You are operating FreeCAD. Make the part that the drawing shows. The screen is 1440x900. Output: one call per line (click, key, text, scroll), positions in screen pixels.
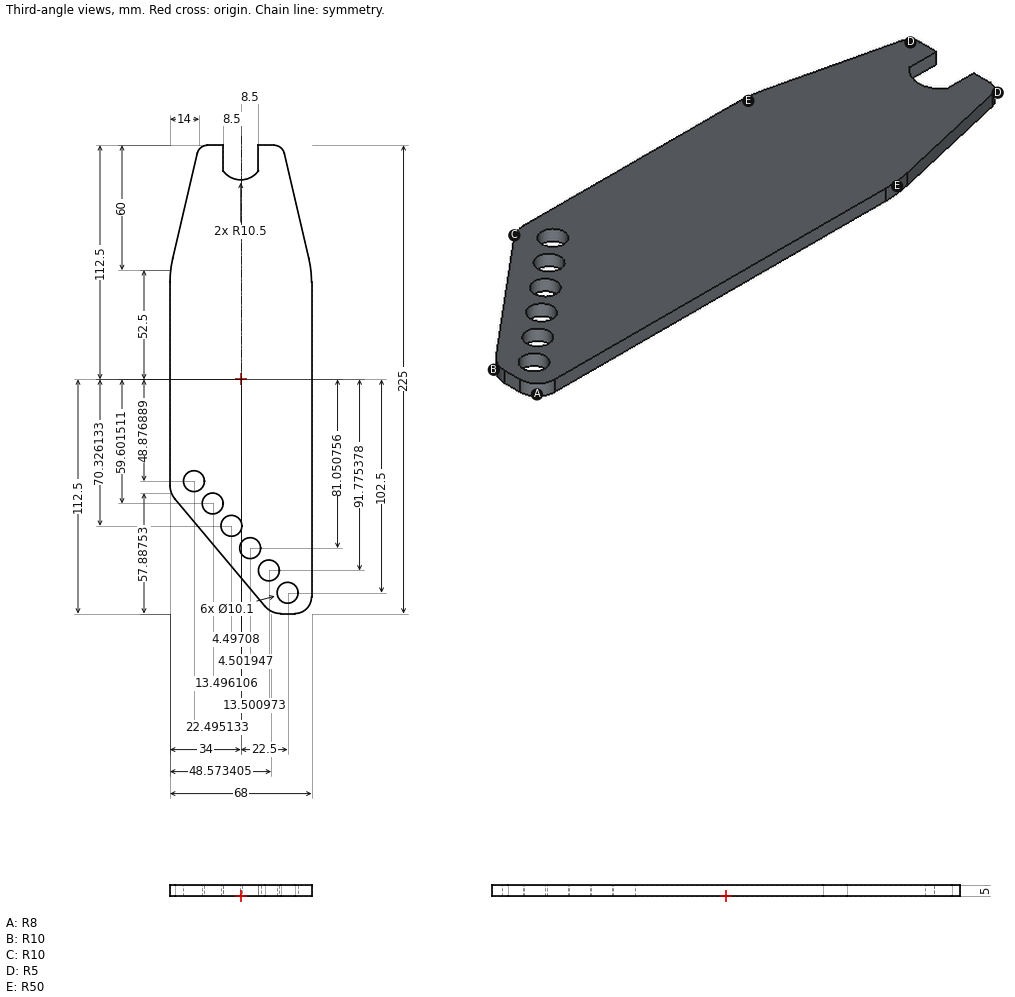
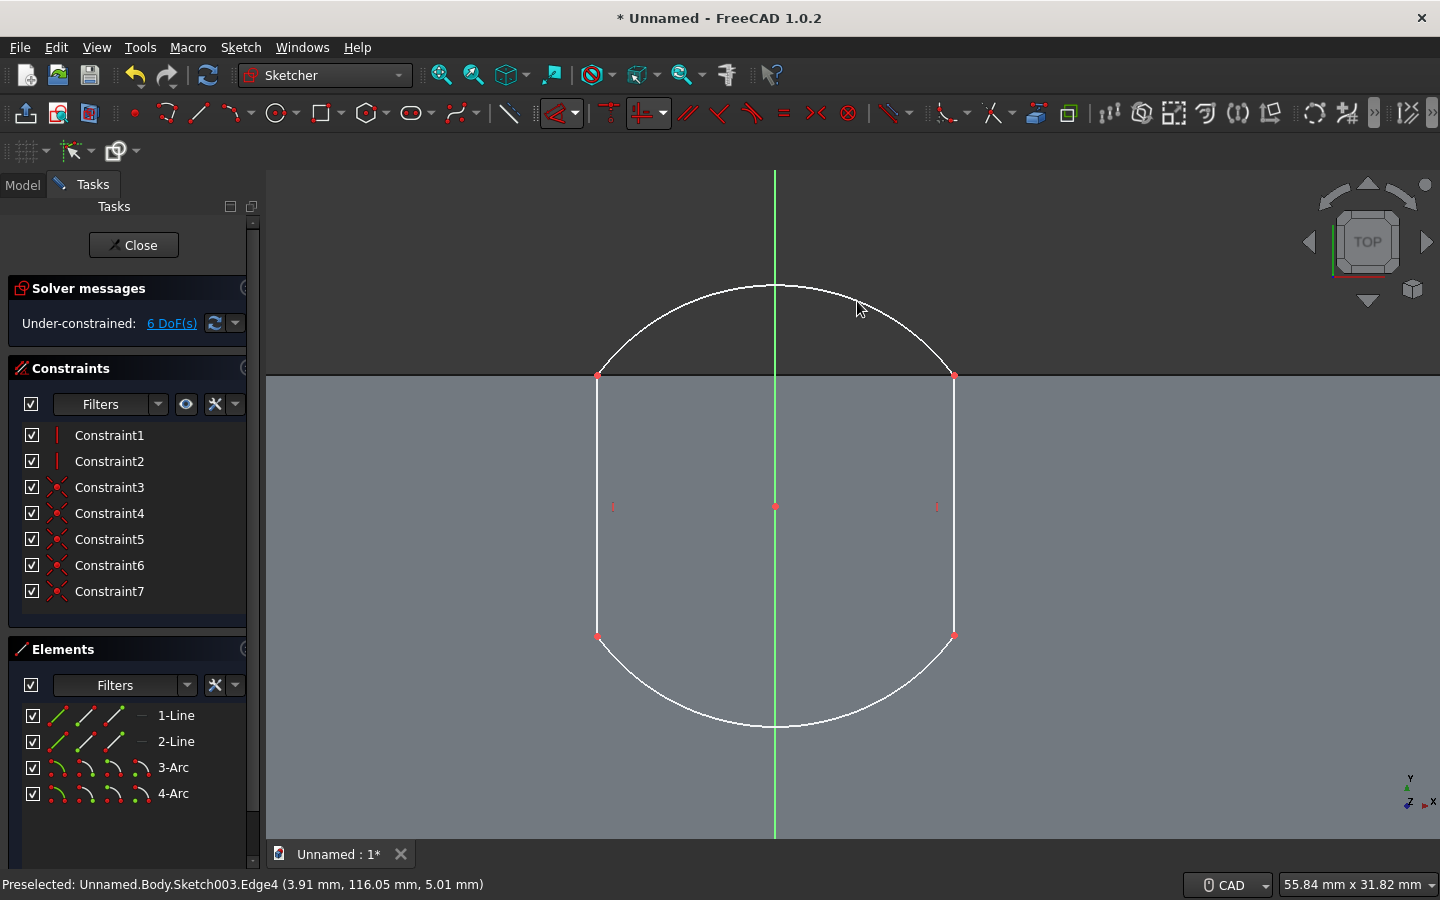
click(694, 711)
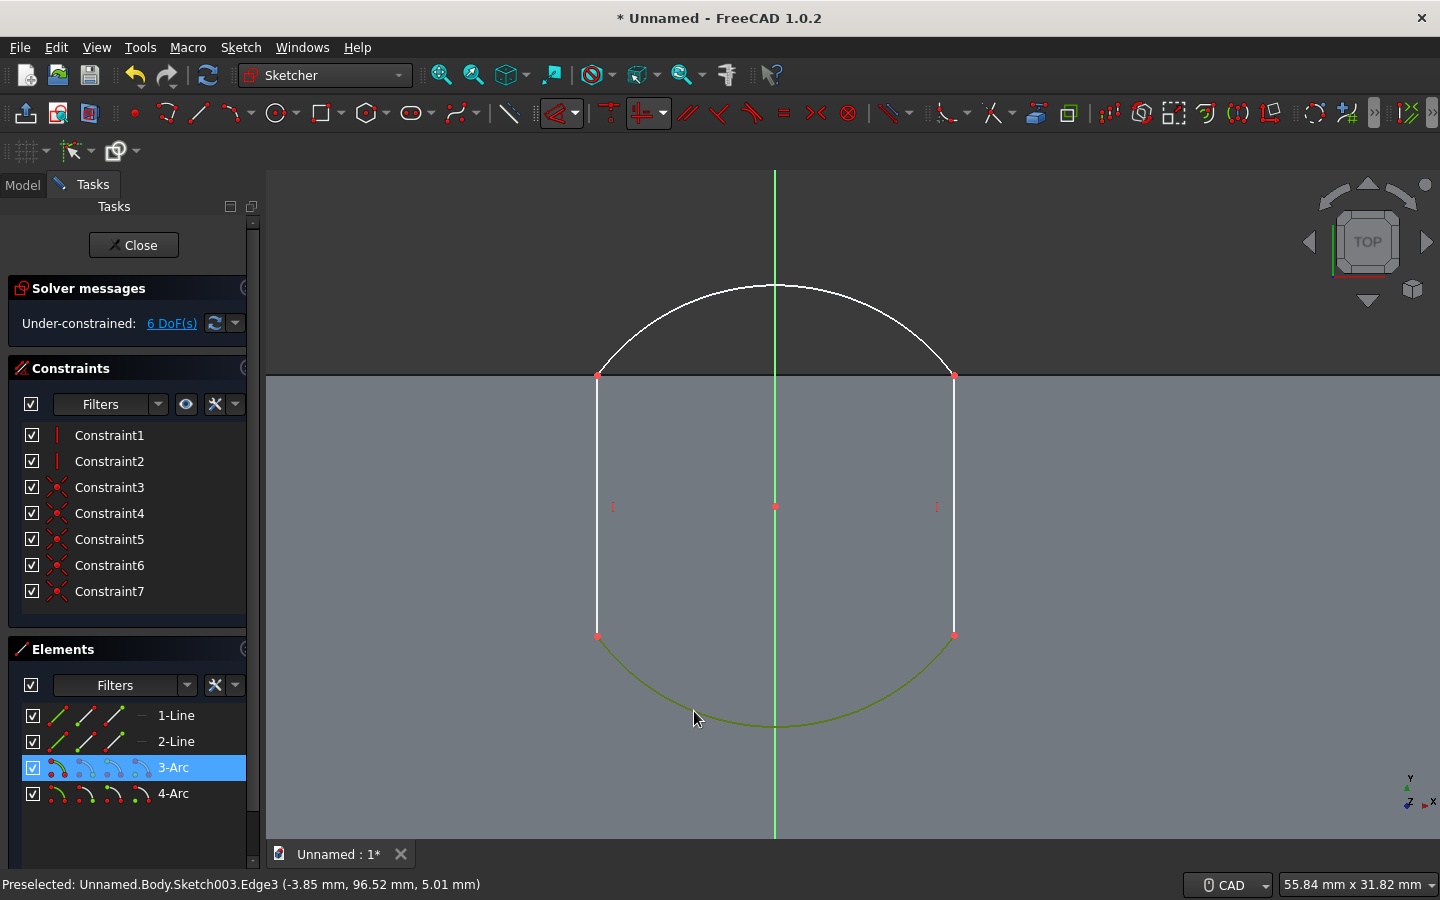
click(857, 301)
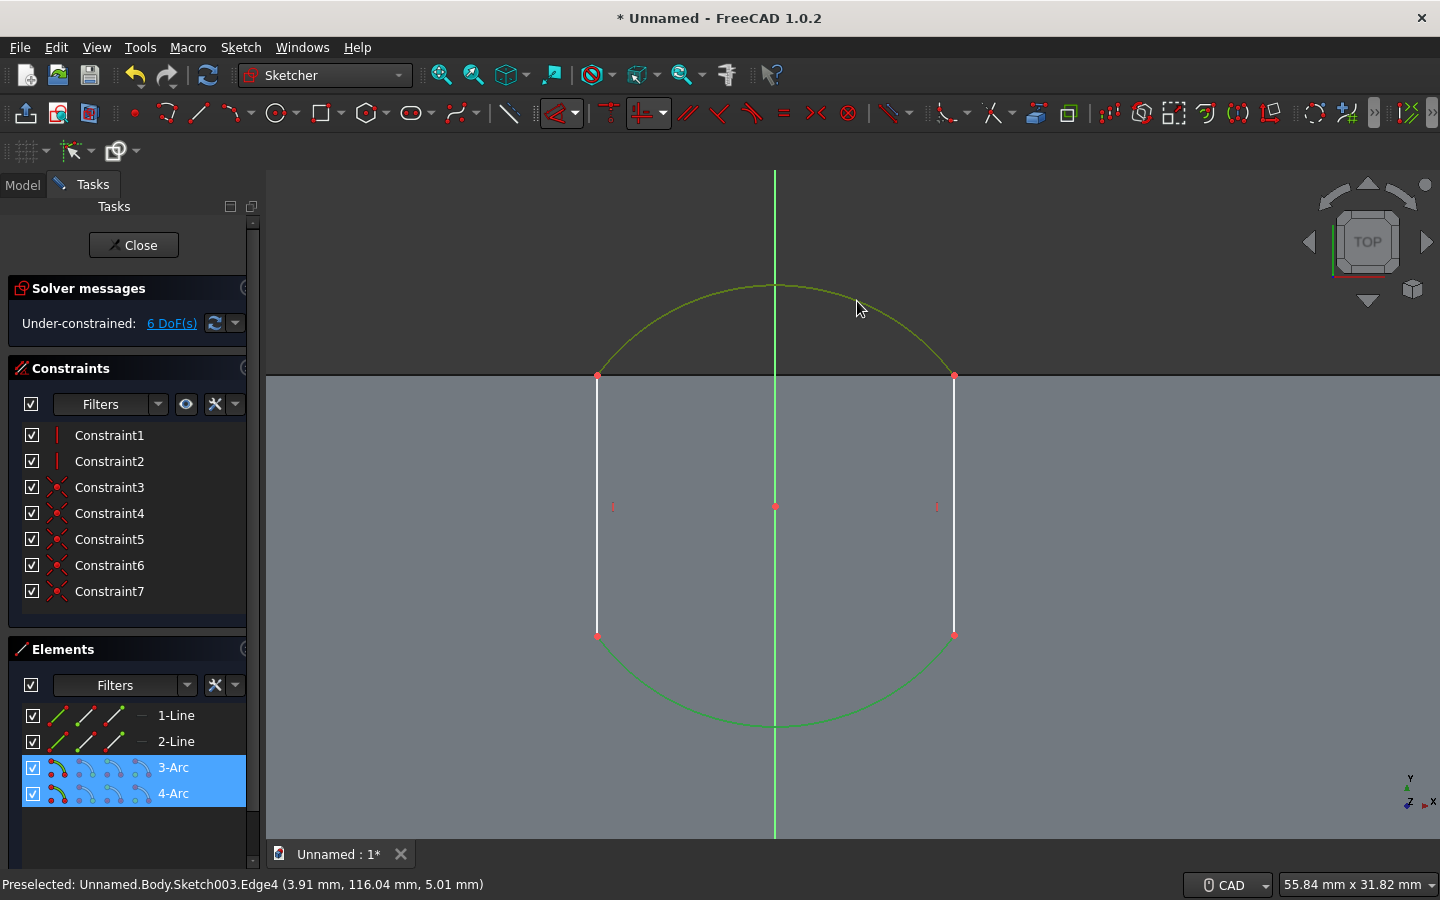
click(784, 114)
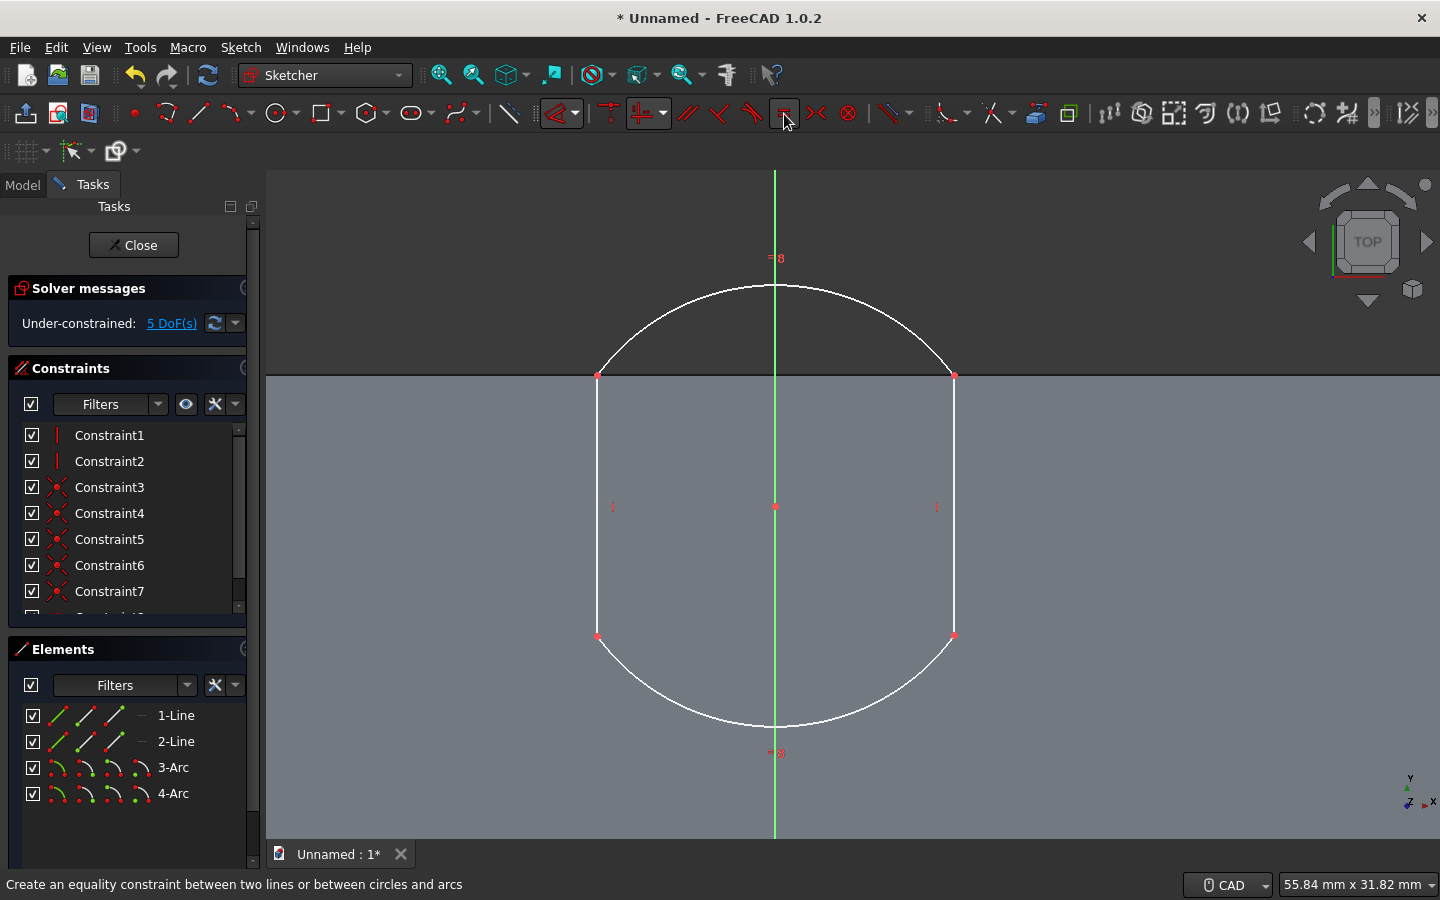
click(775, 506)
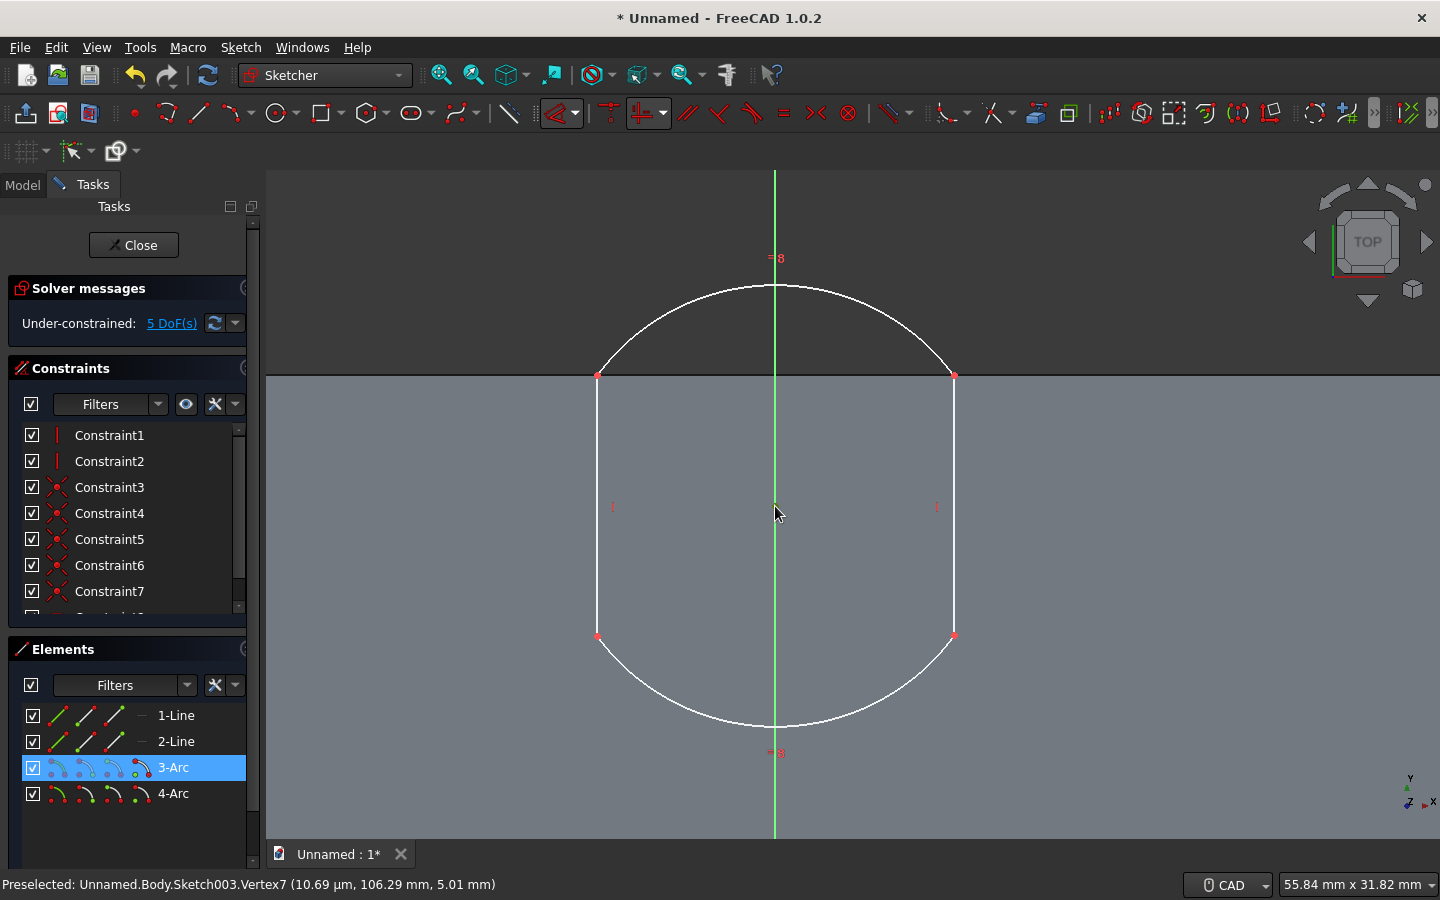
click(775, 767)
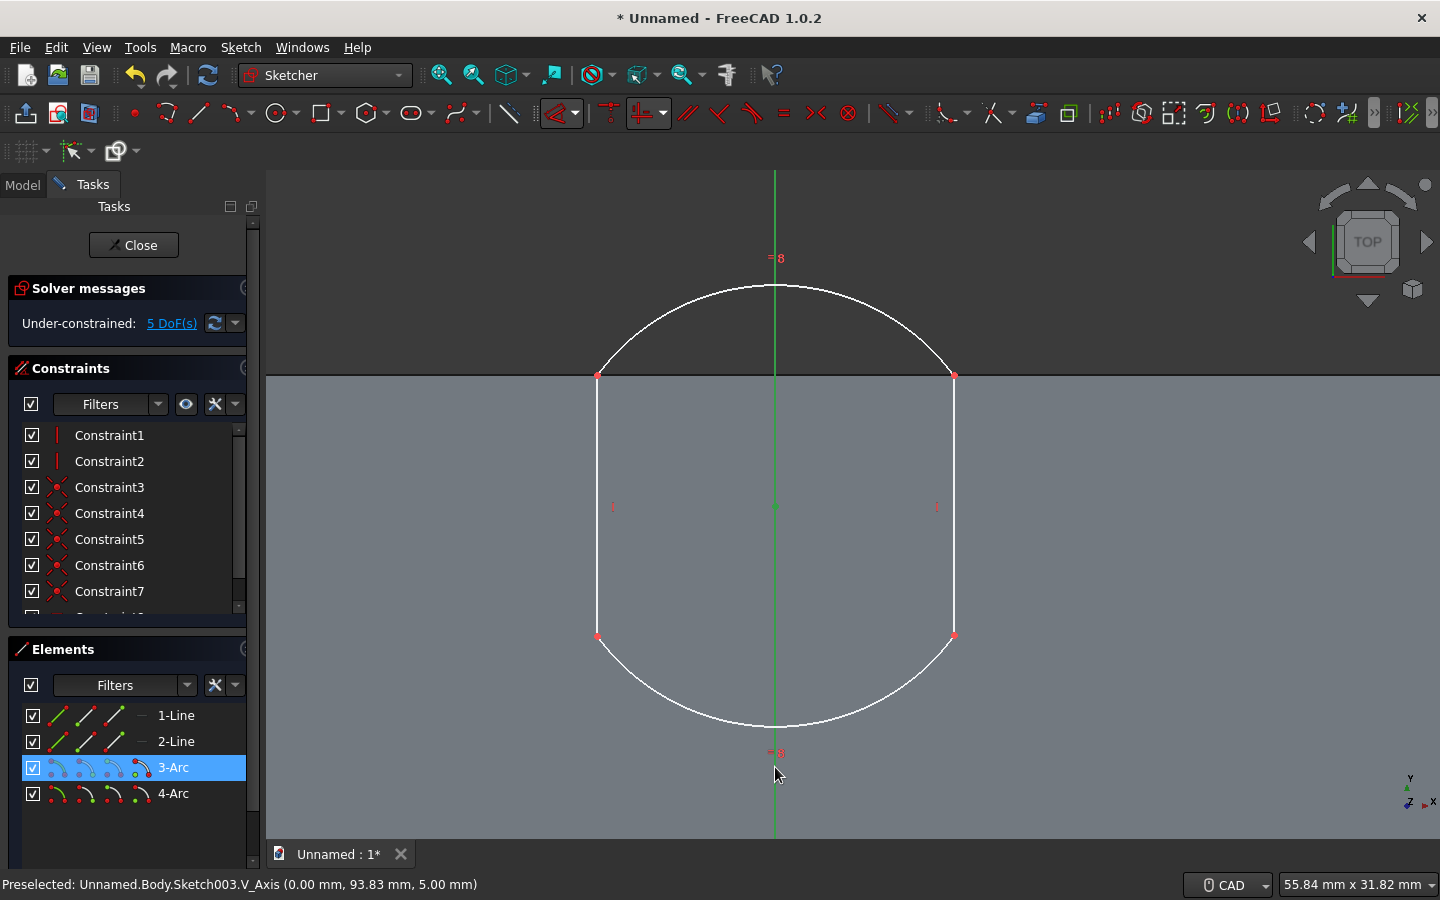
key(c)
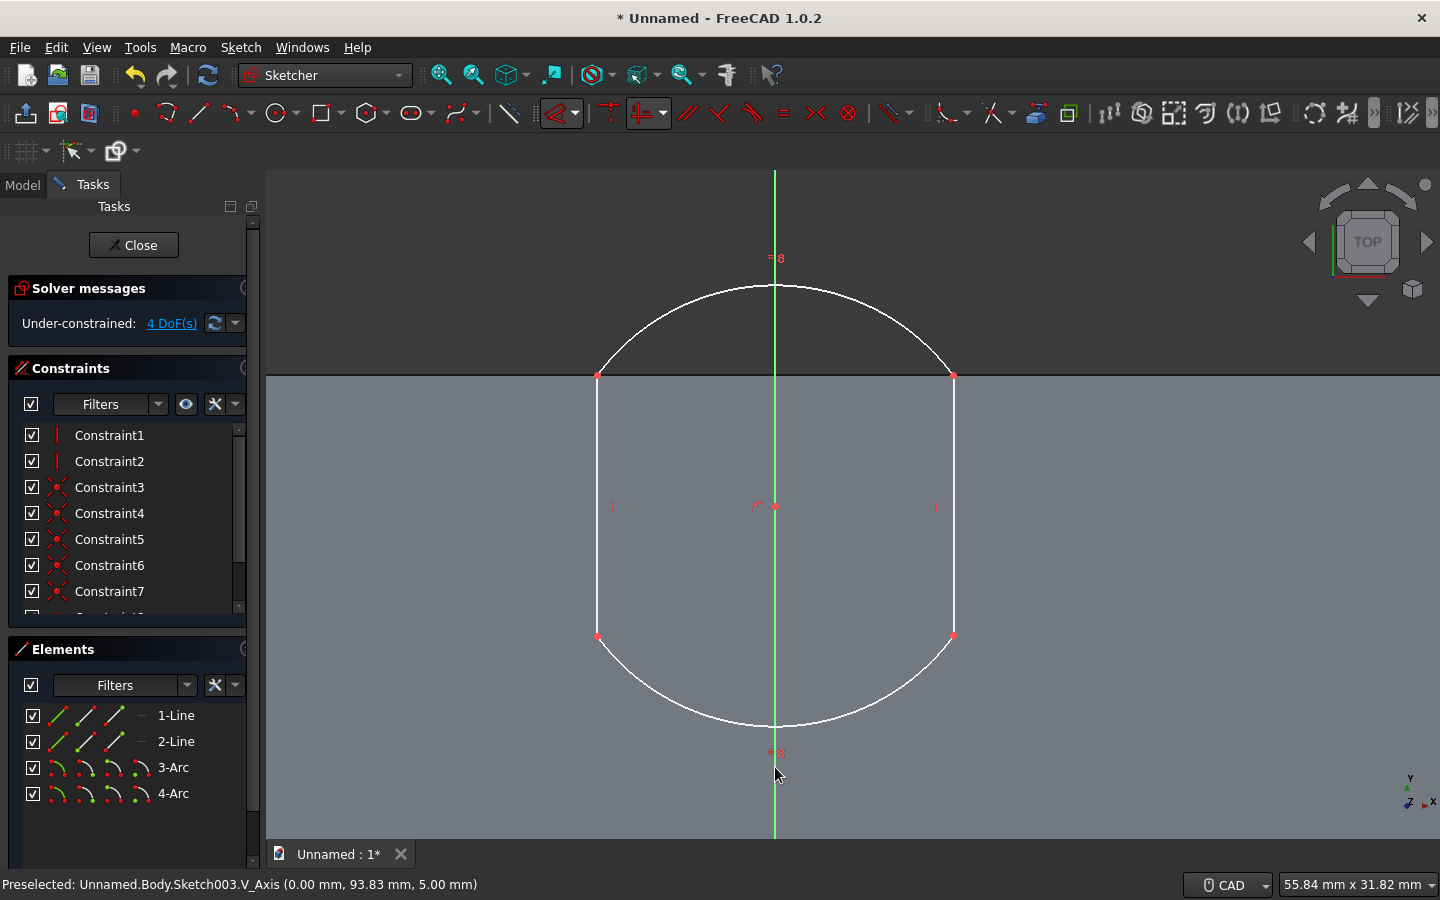
click(694, 711)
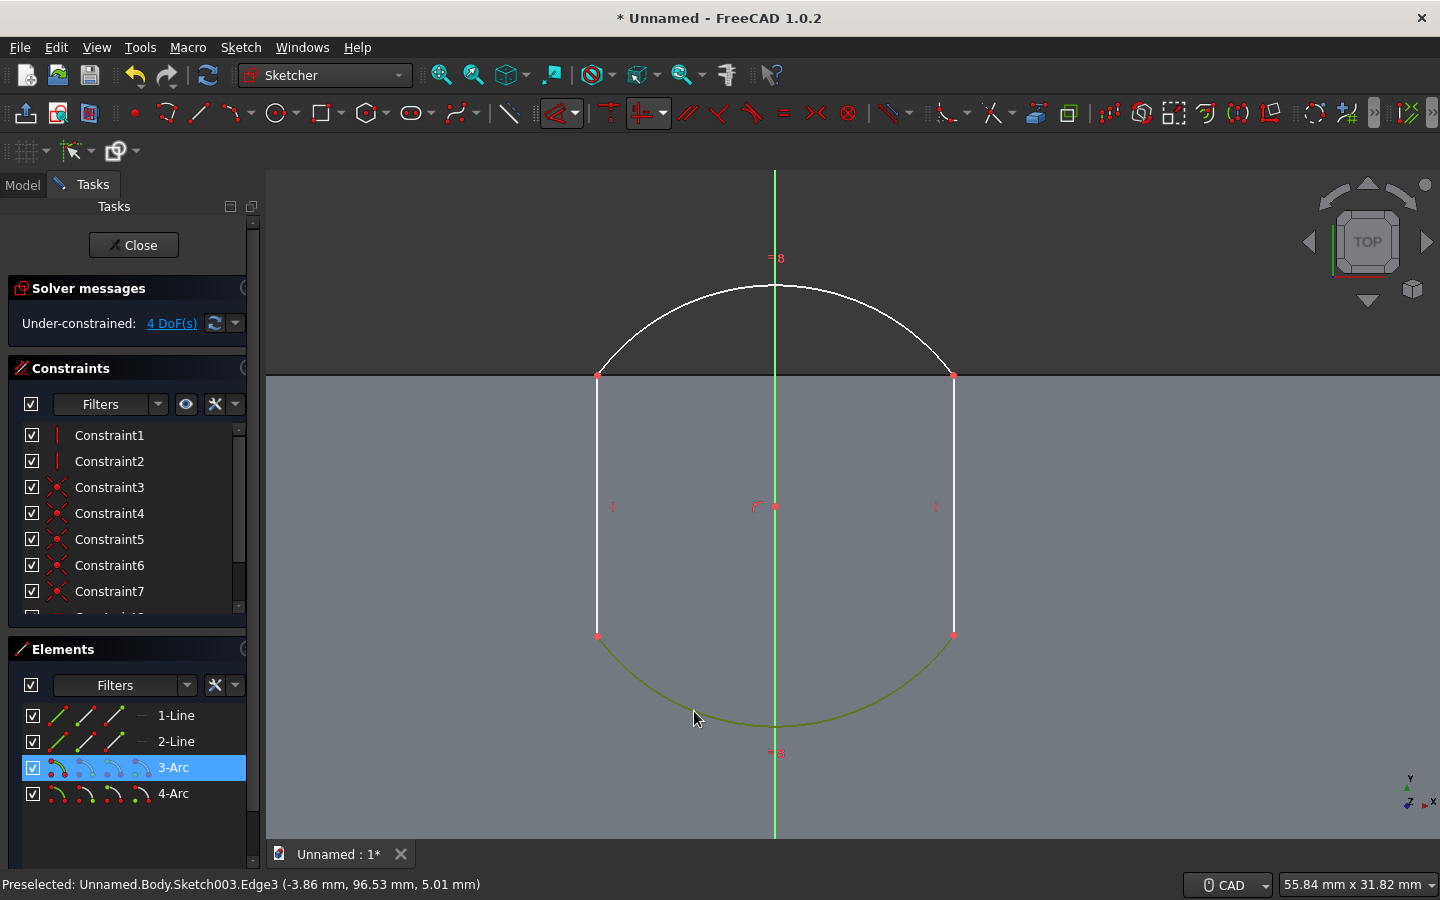
click(578, 114)